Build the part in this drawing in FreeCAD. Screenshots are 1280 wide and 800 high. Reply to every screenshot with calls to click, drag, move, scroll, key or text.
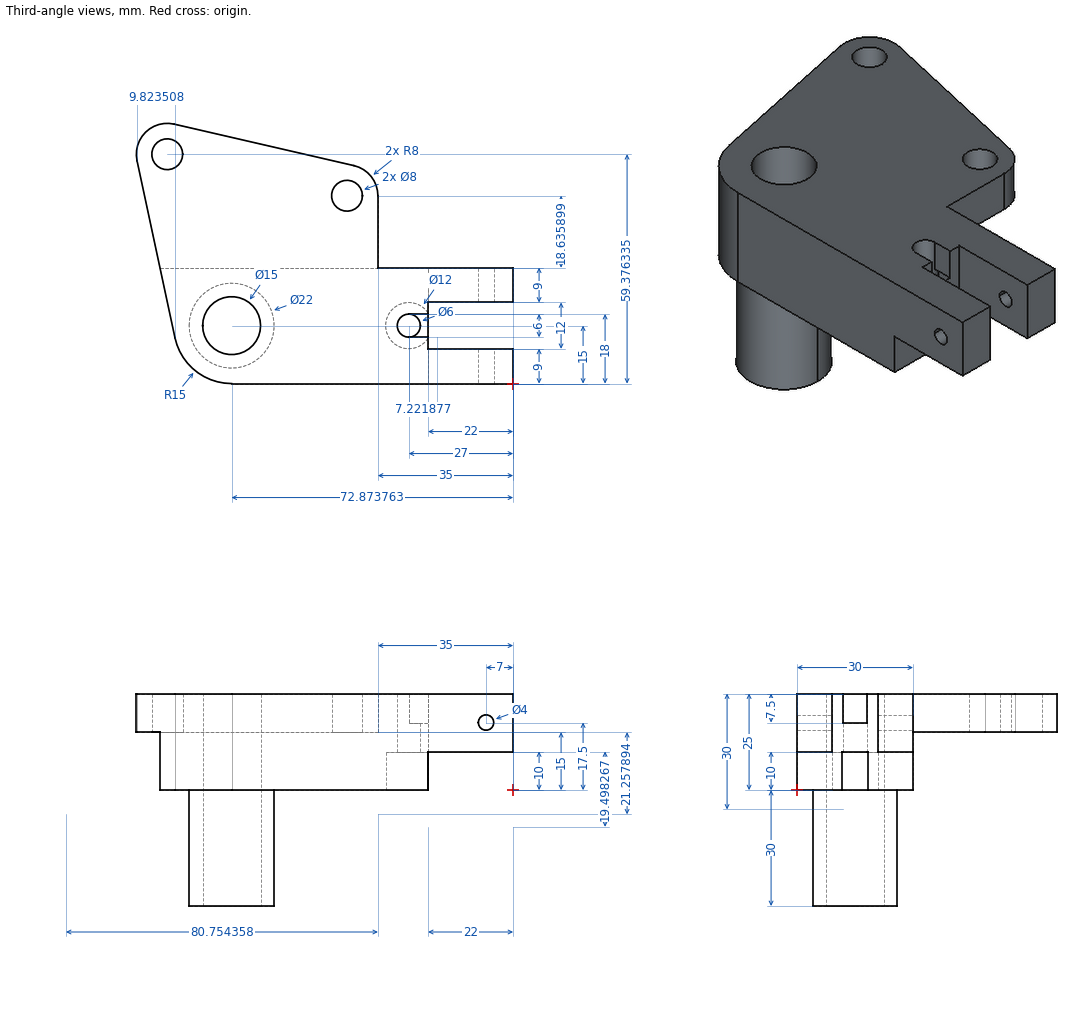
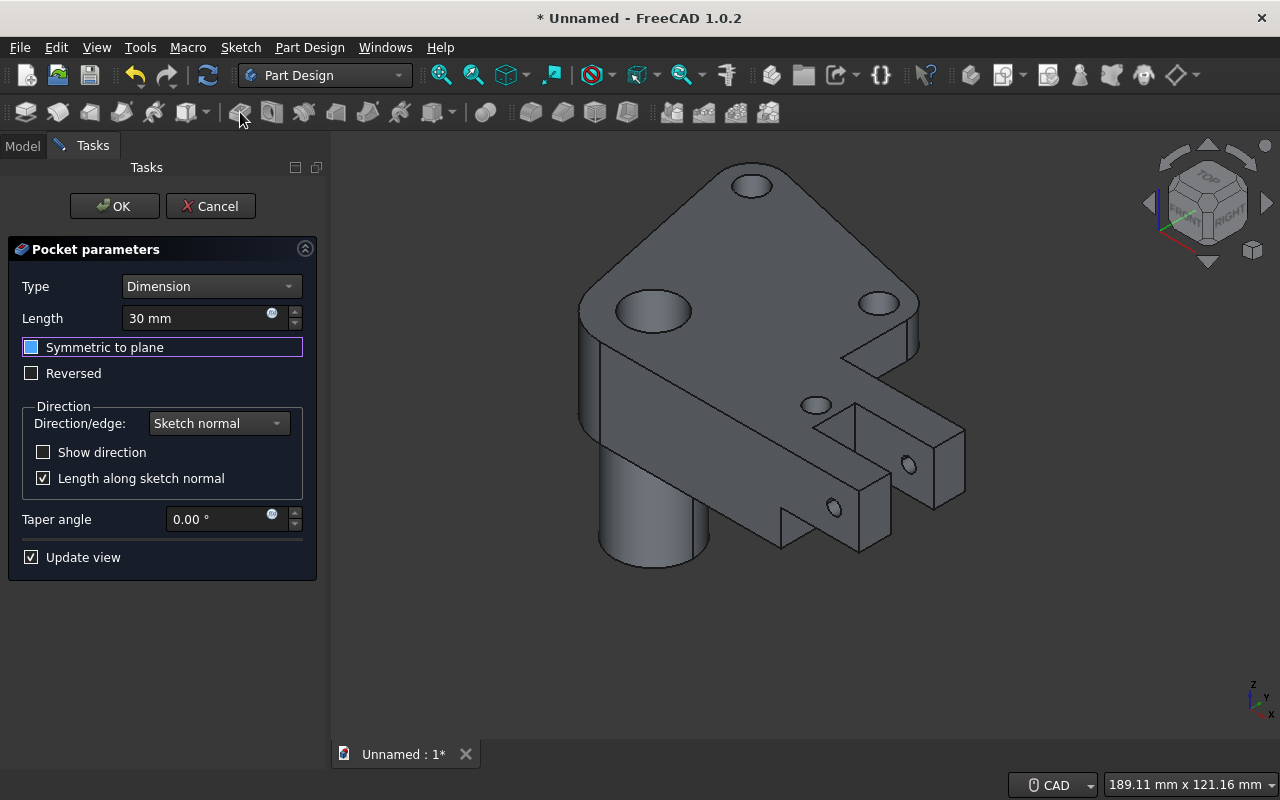
click(115, 206)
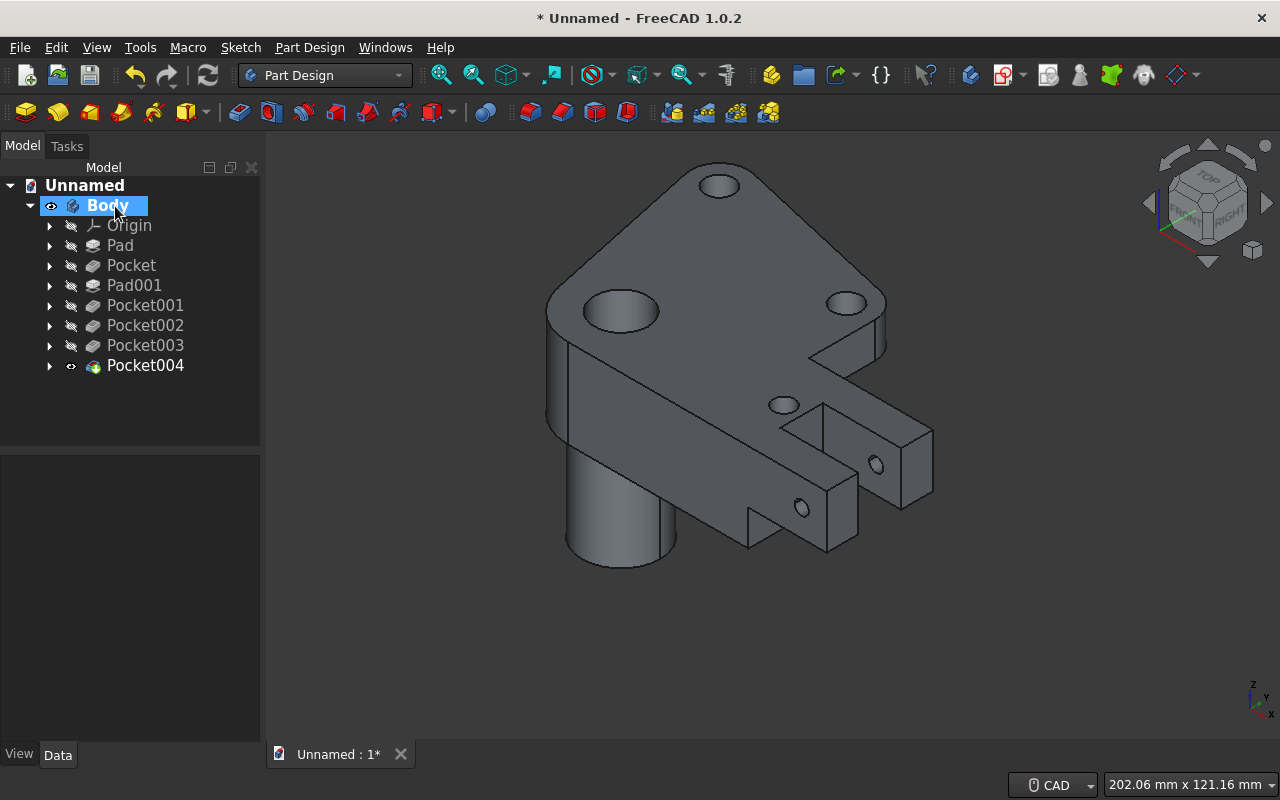
click(708, 245)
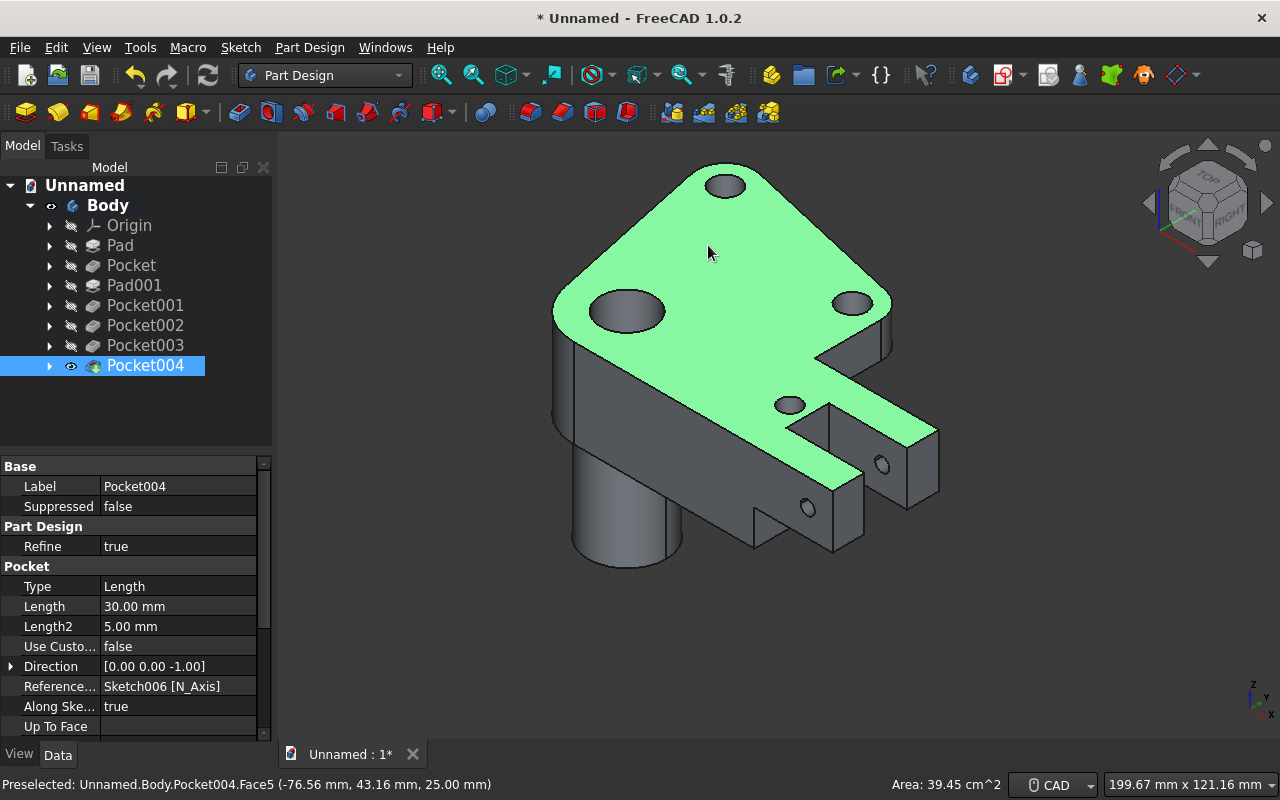
click(1004, 76)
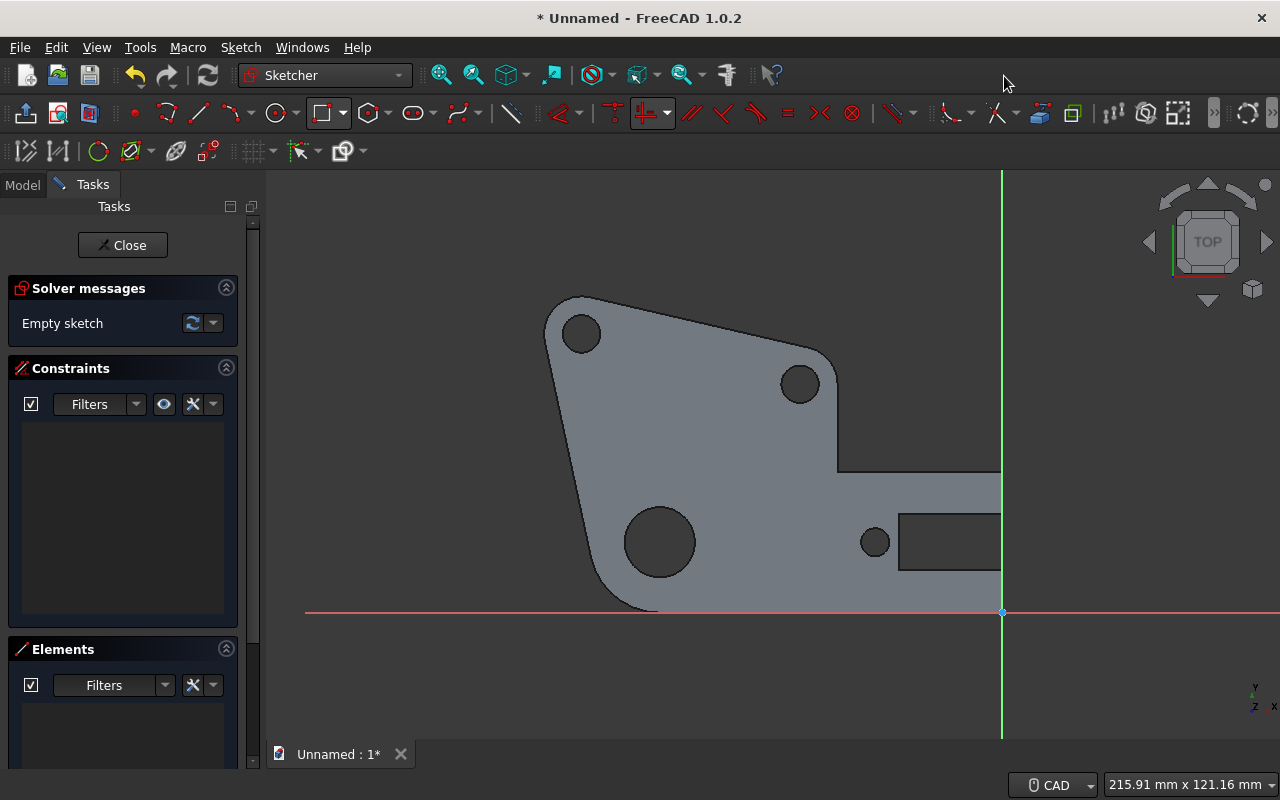
scroll(907, 549, up, 13)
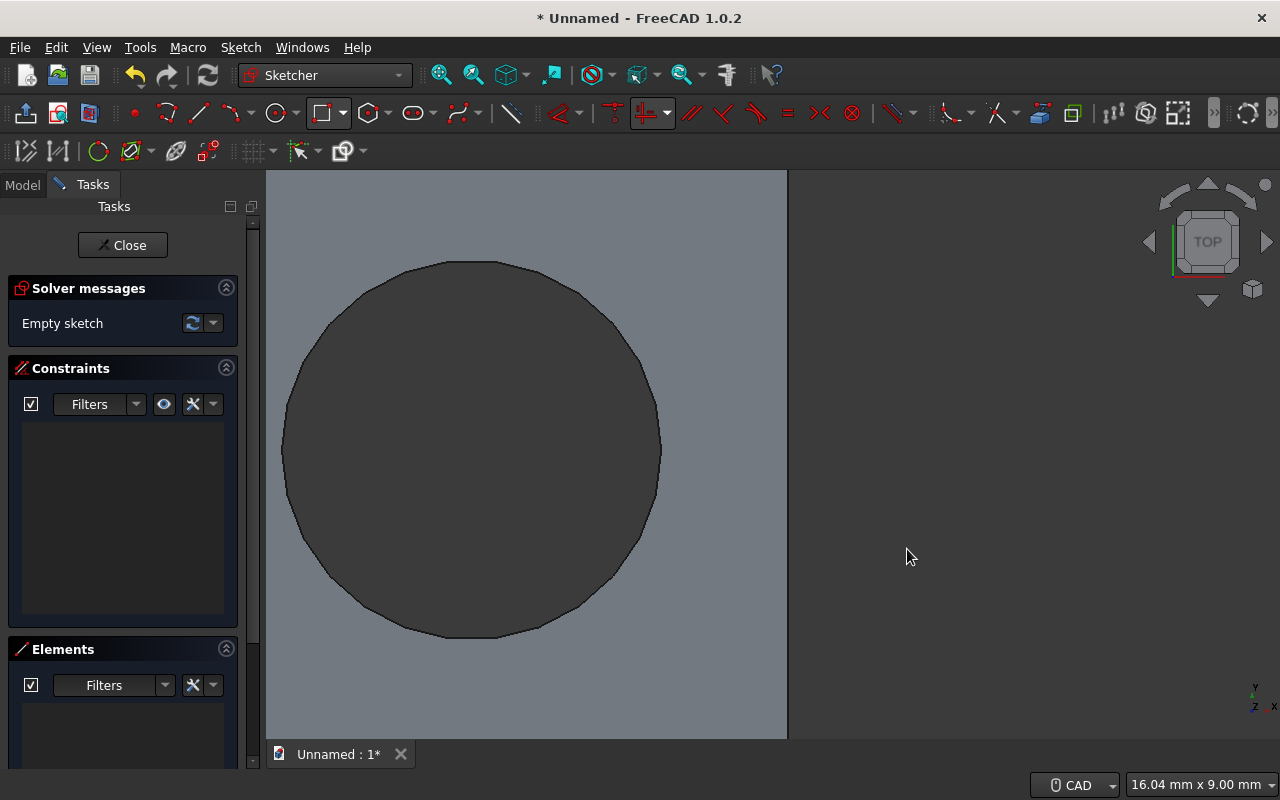
key(g)
key(r)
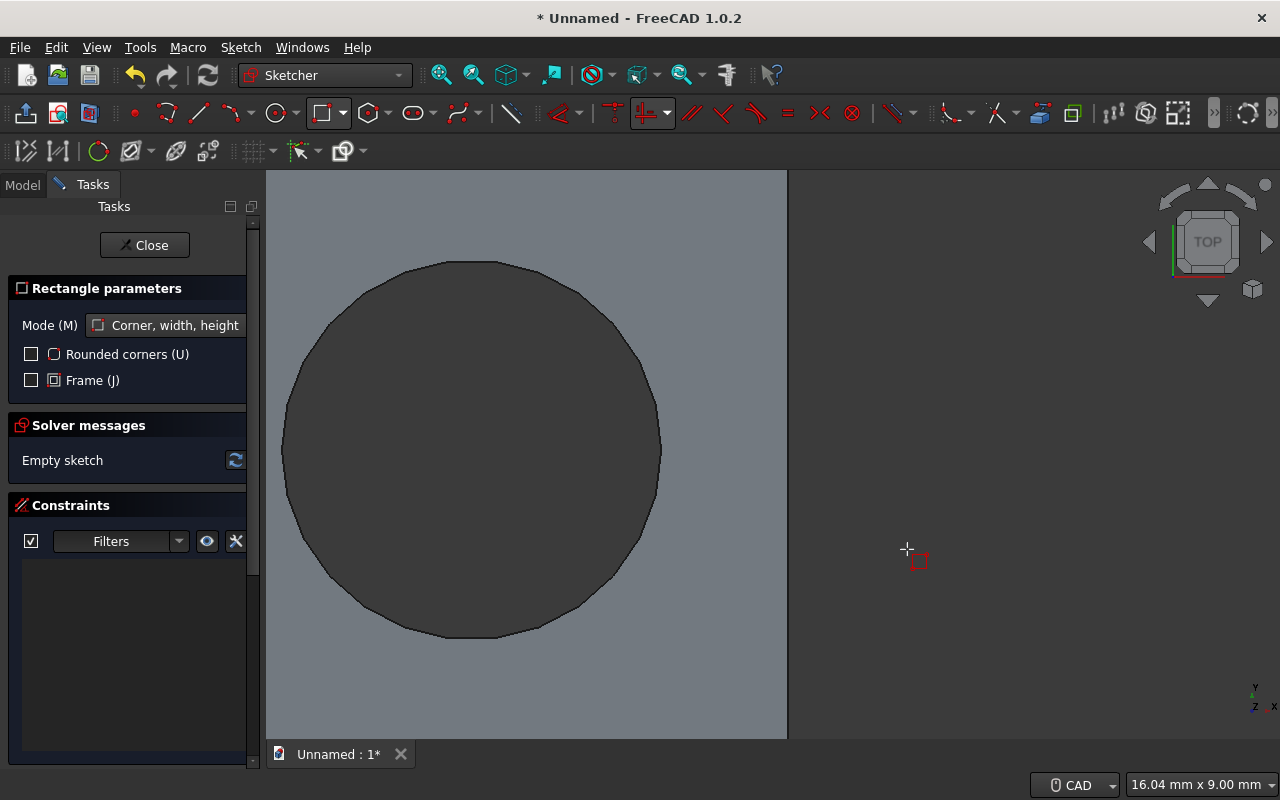
click(472, 260)
click(928, 640)
key(Escape)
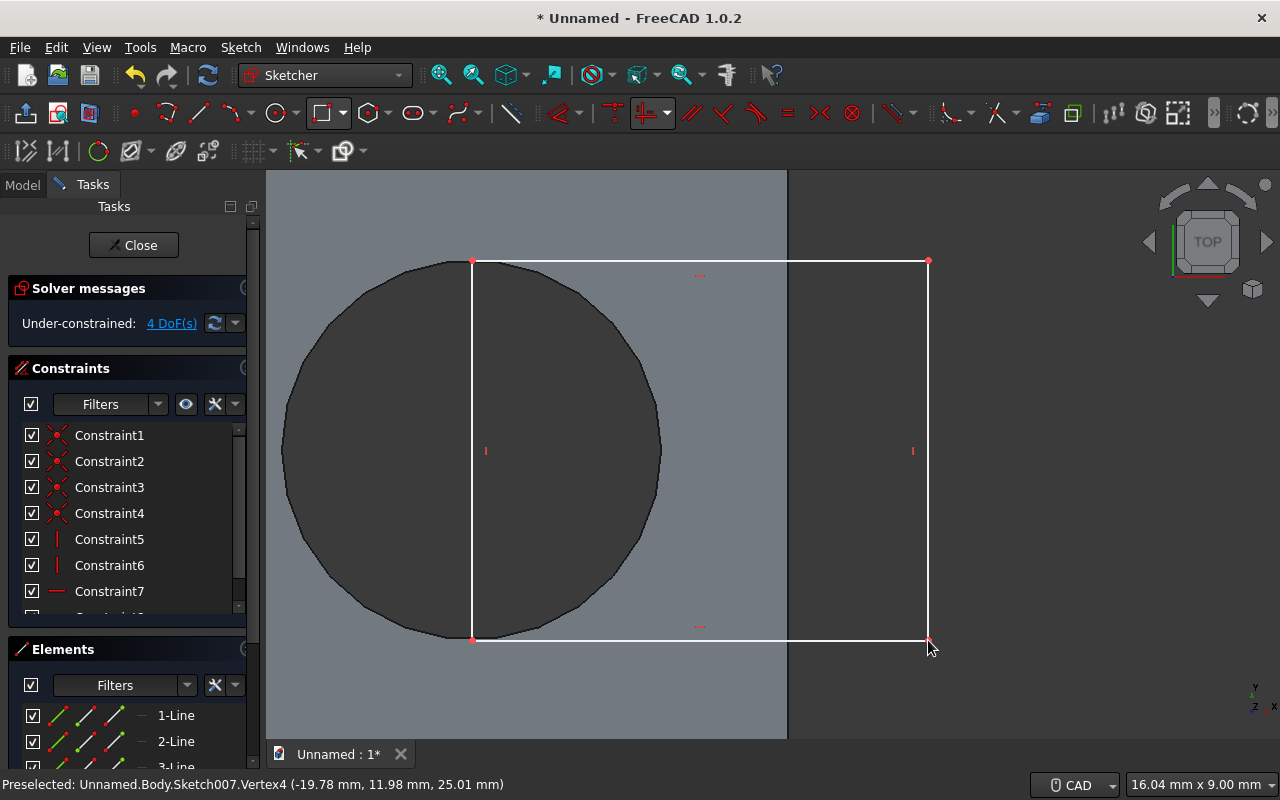
click(558, 114)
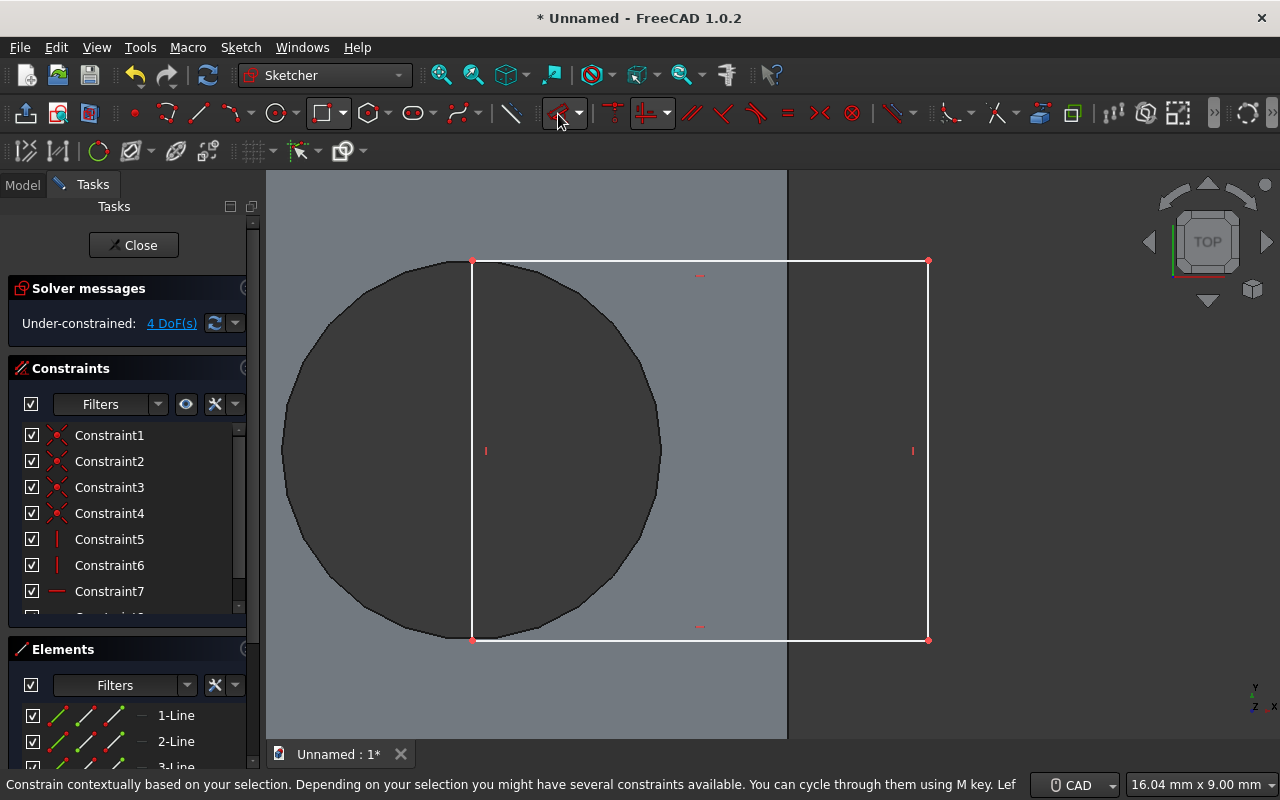
click(472, 375)
click(438, 451)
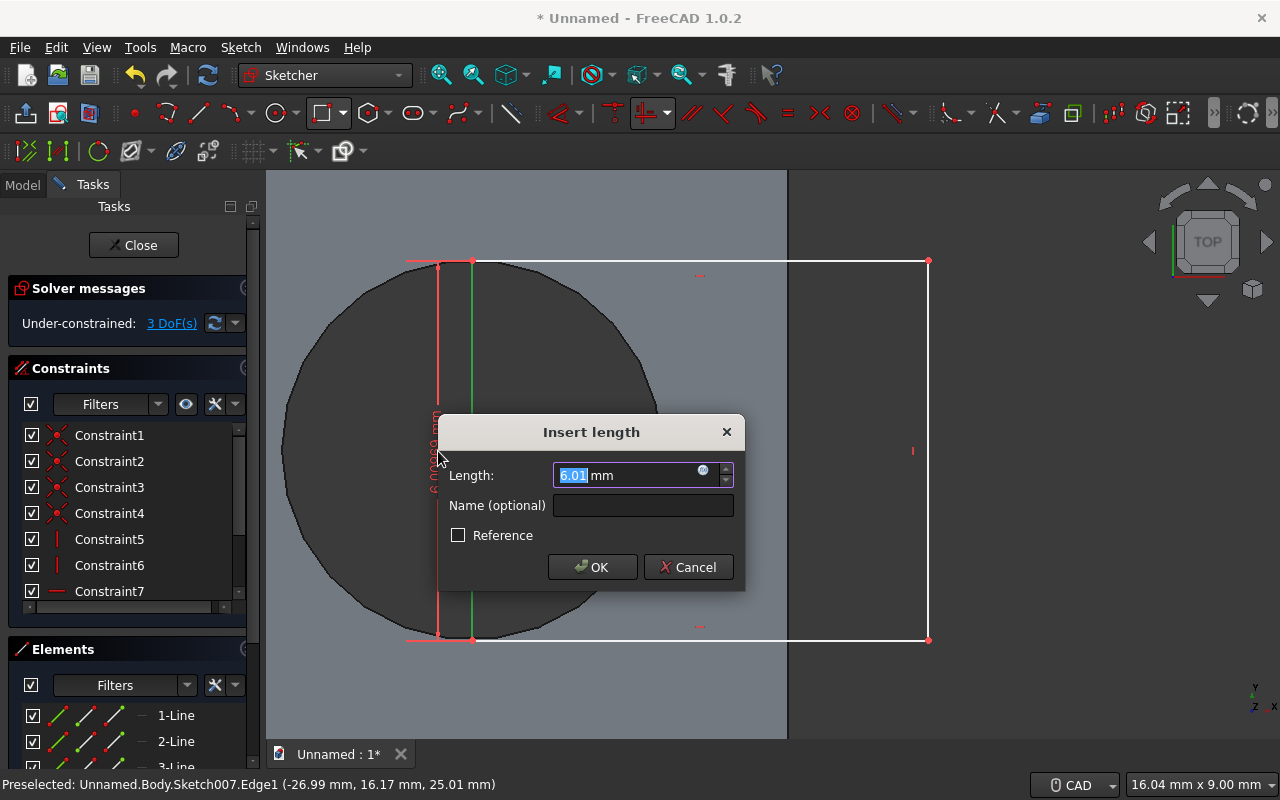
text(6)
key(Return)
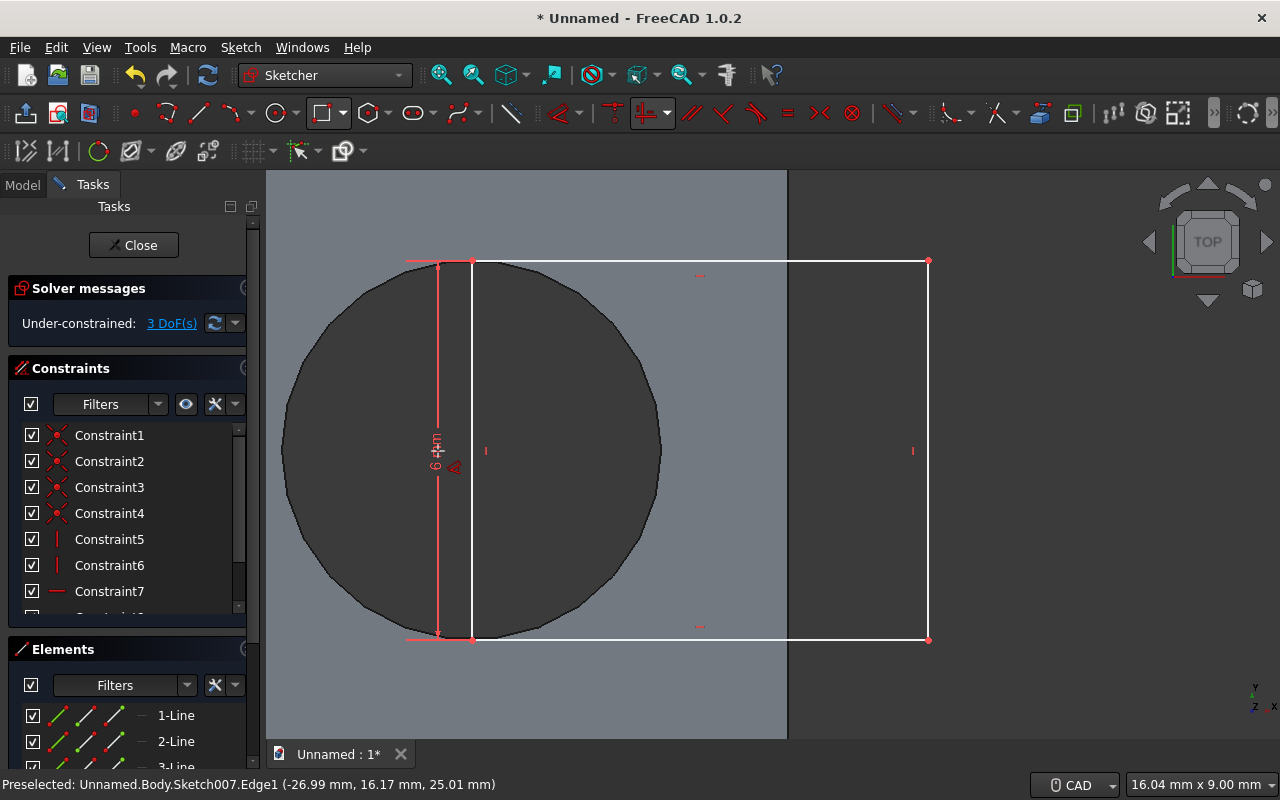
click(472, 261)
click(794, 227)